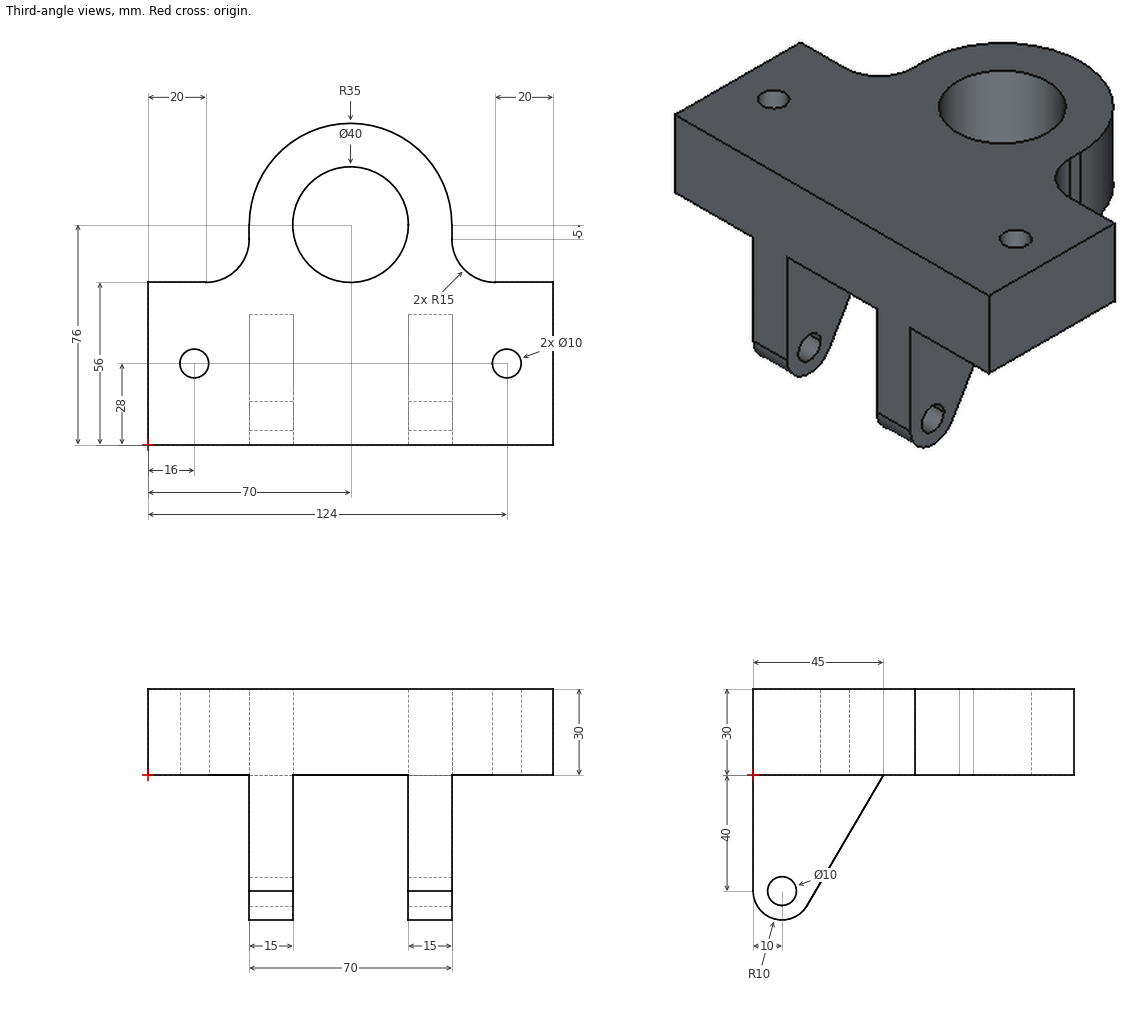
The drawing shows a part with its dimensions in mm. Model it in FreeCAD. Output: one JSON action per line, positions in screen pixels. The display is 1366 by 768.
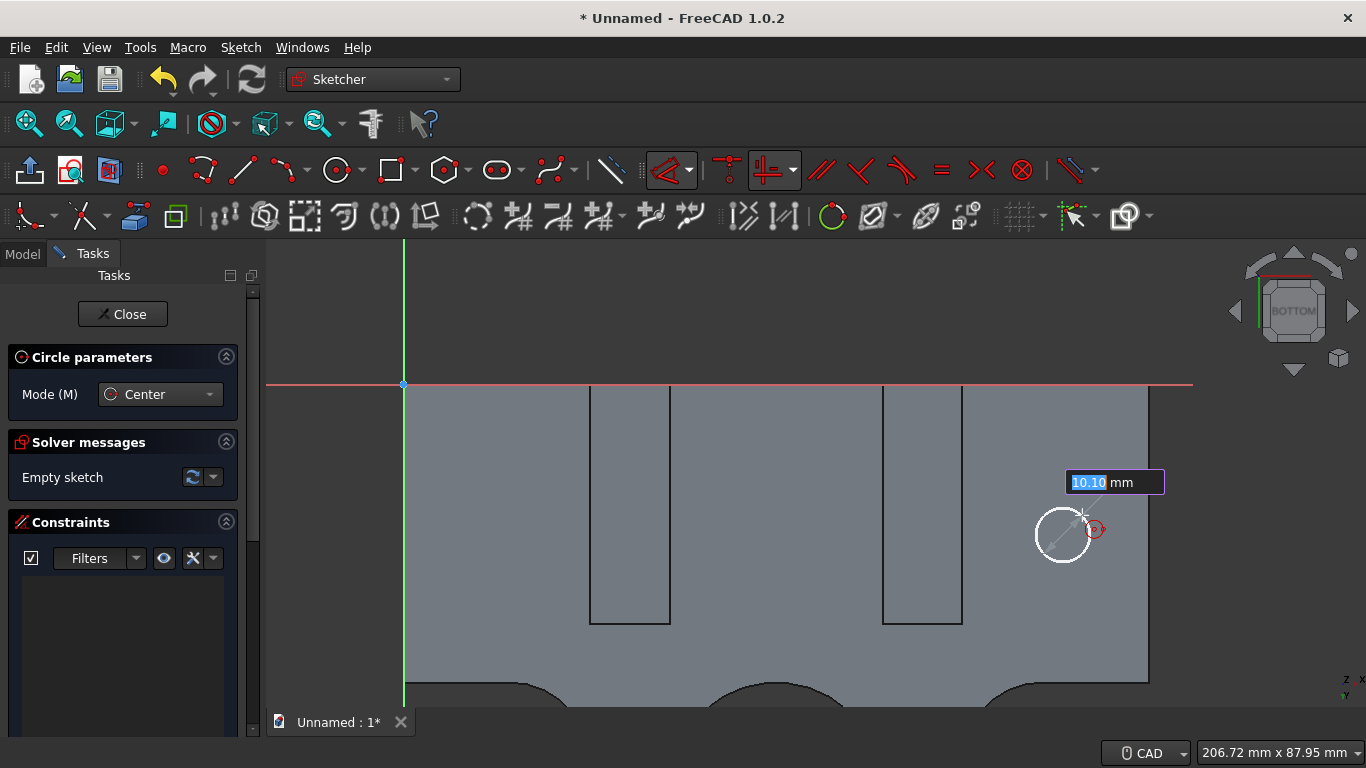
{"action": "type", "text": "10"}
{"action": "key", "text": "Return"}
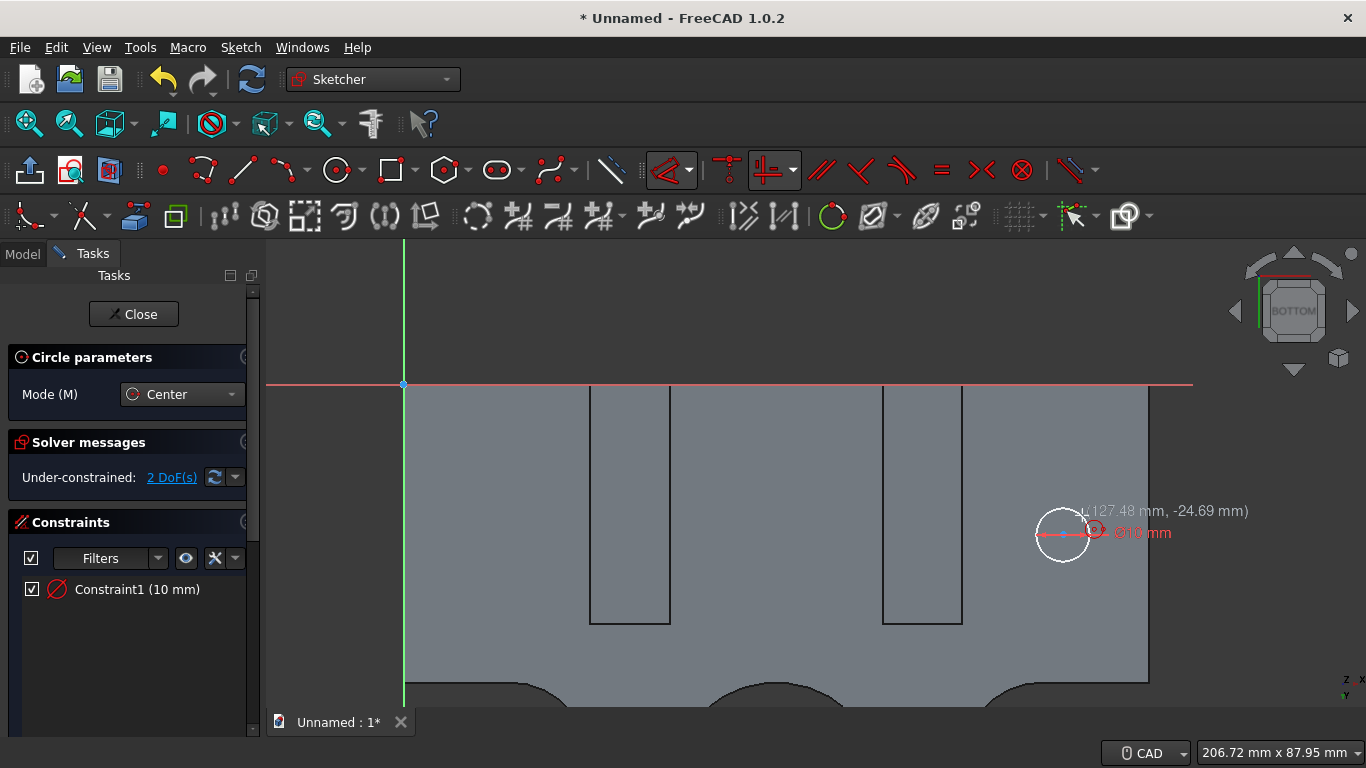
{"action": "left_click", "coordinate": [489, 534]}
{"action": "mouse_move", "coordinate": [508, 515]}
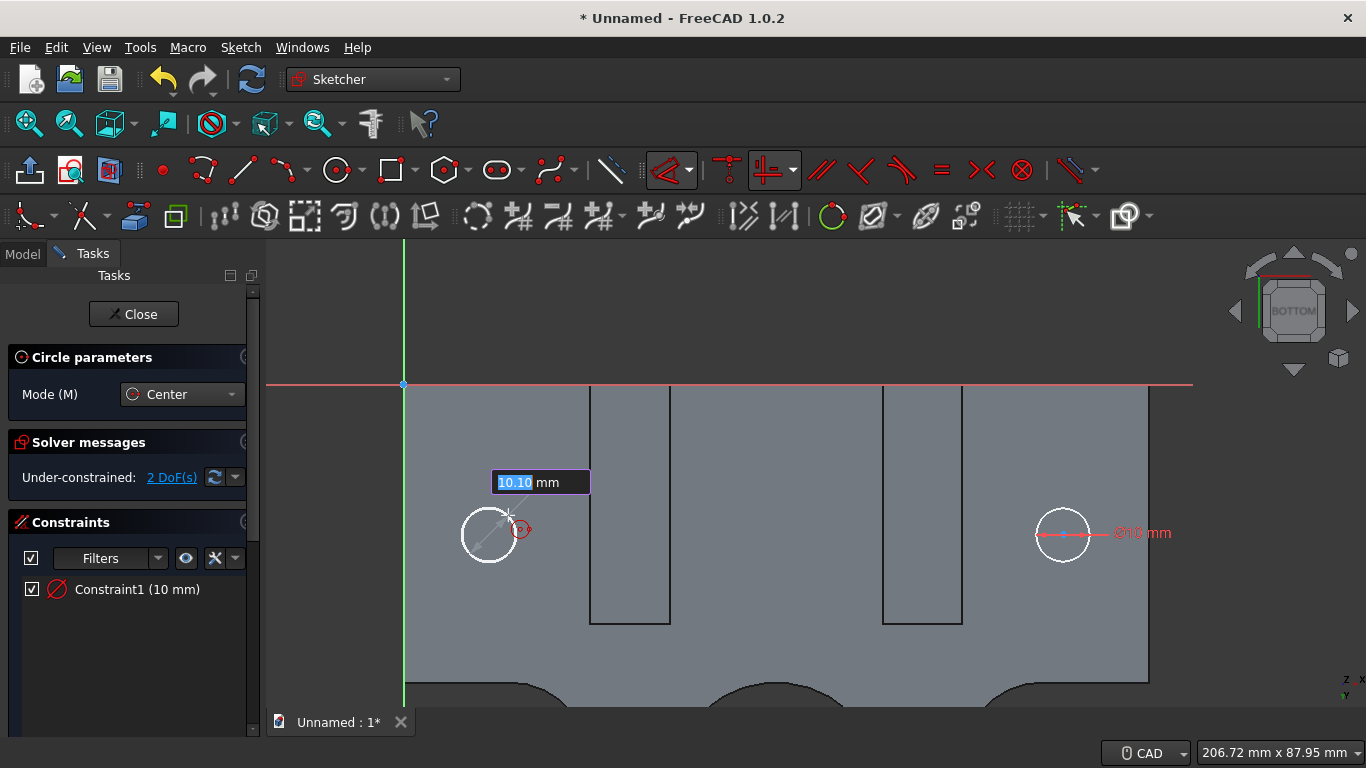
{"action": "type", "text": "10"}
{"action": "key", "text": "Return"}
{"action": "key", "text": "Escape"}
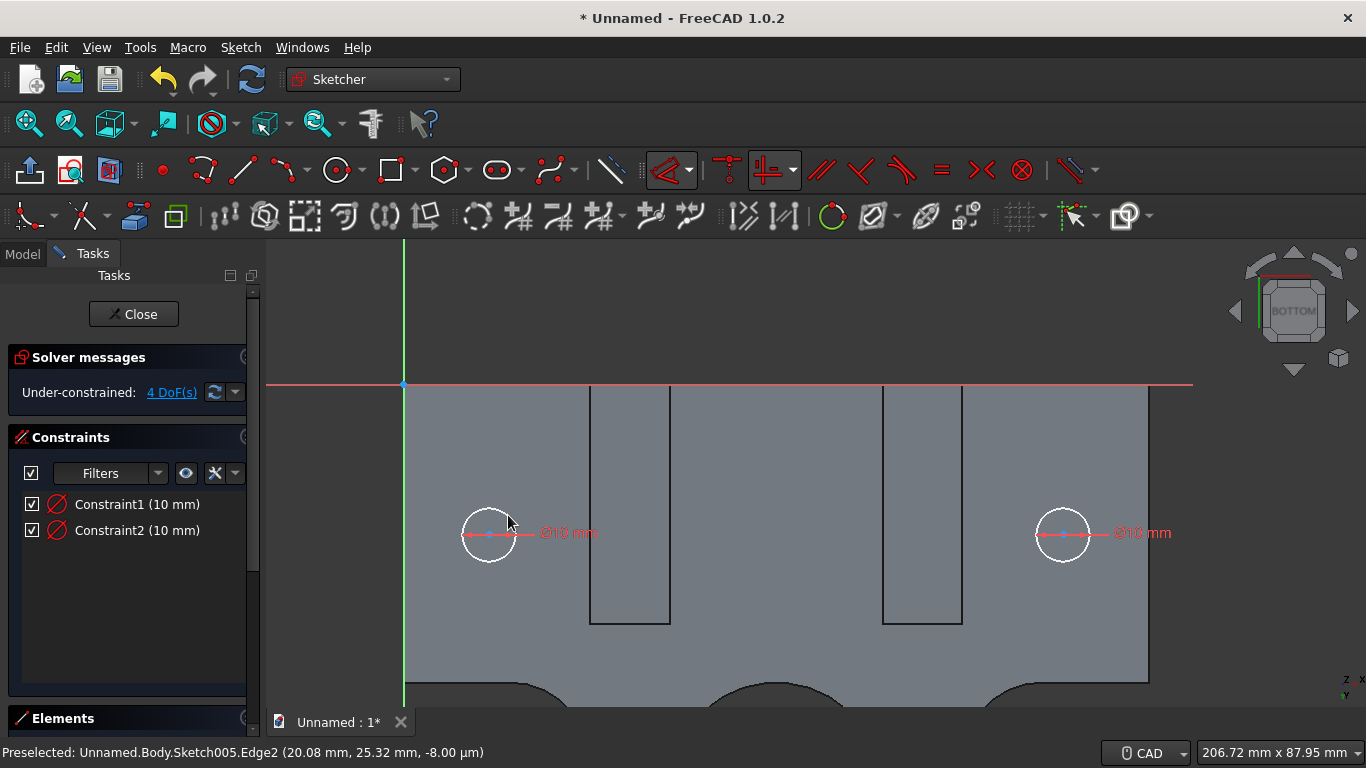
{"action": "left_click", "coordinate": [1063, 535]}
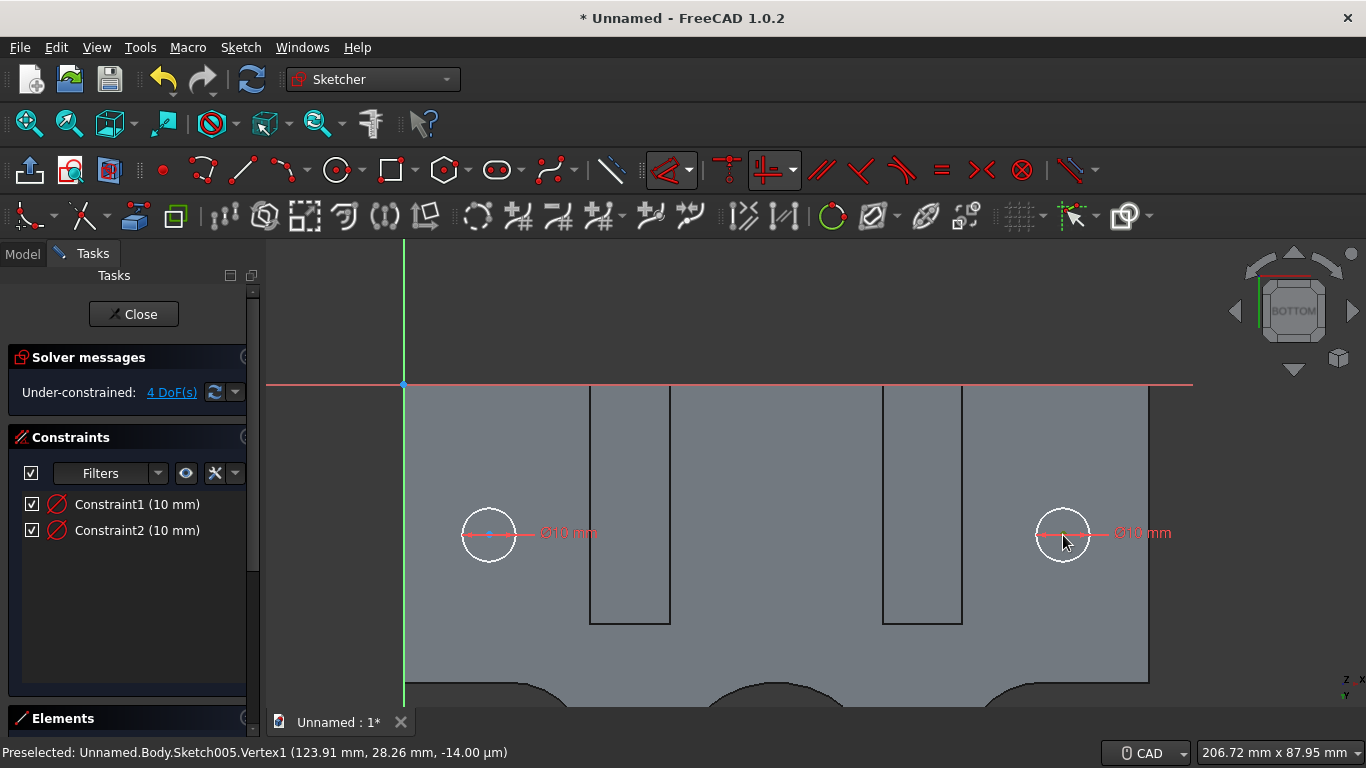
{"action": "left_click", "coordinate": [489, 535]}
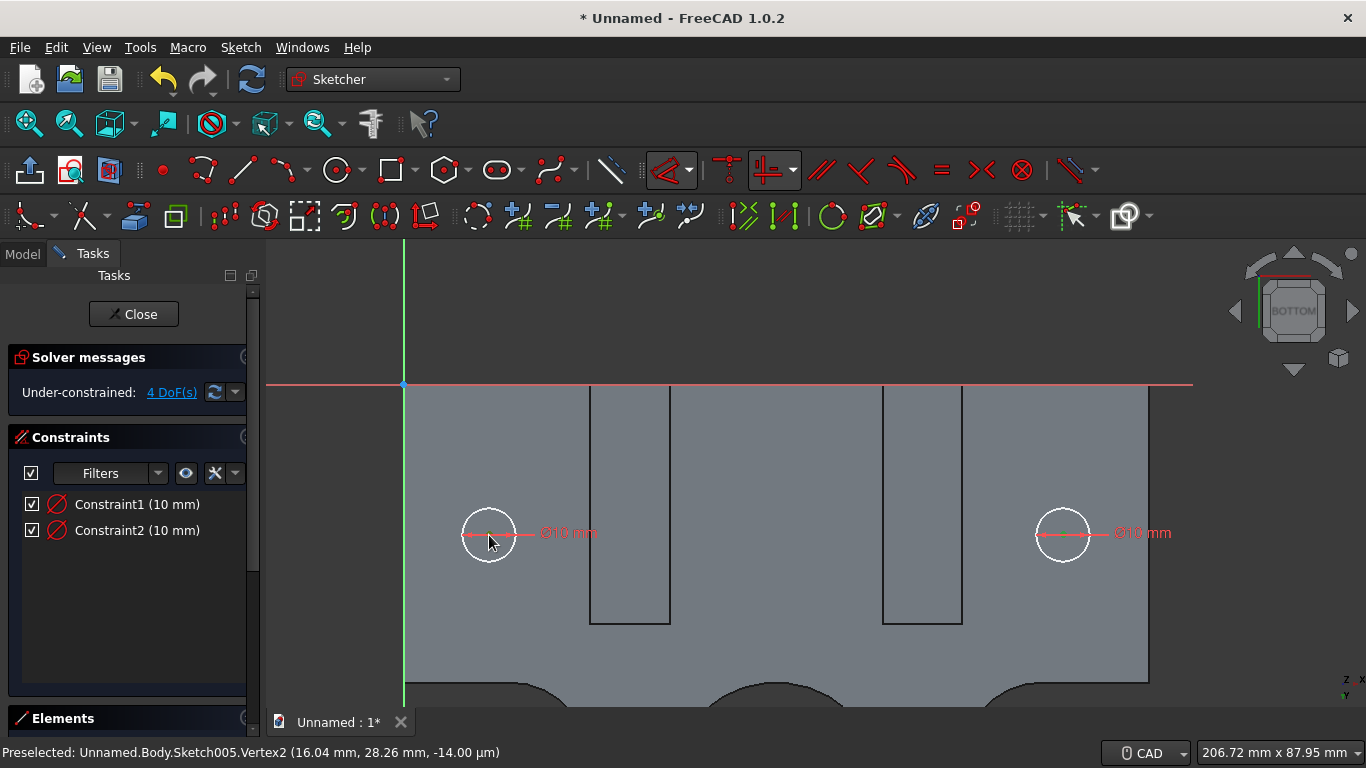
{"action": "key", "text": "h"}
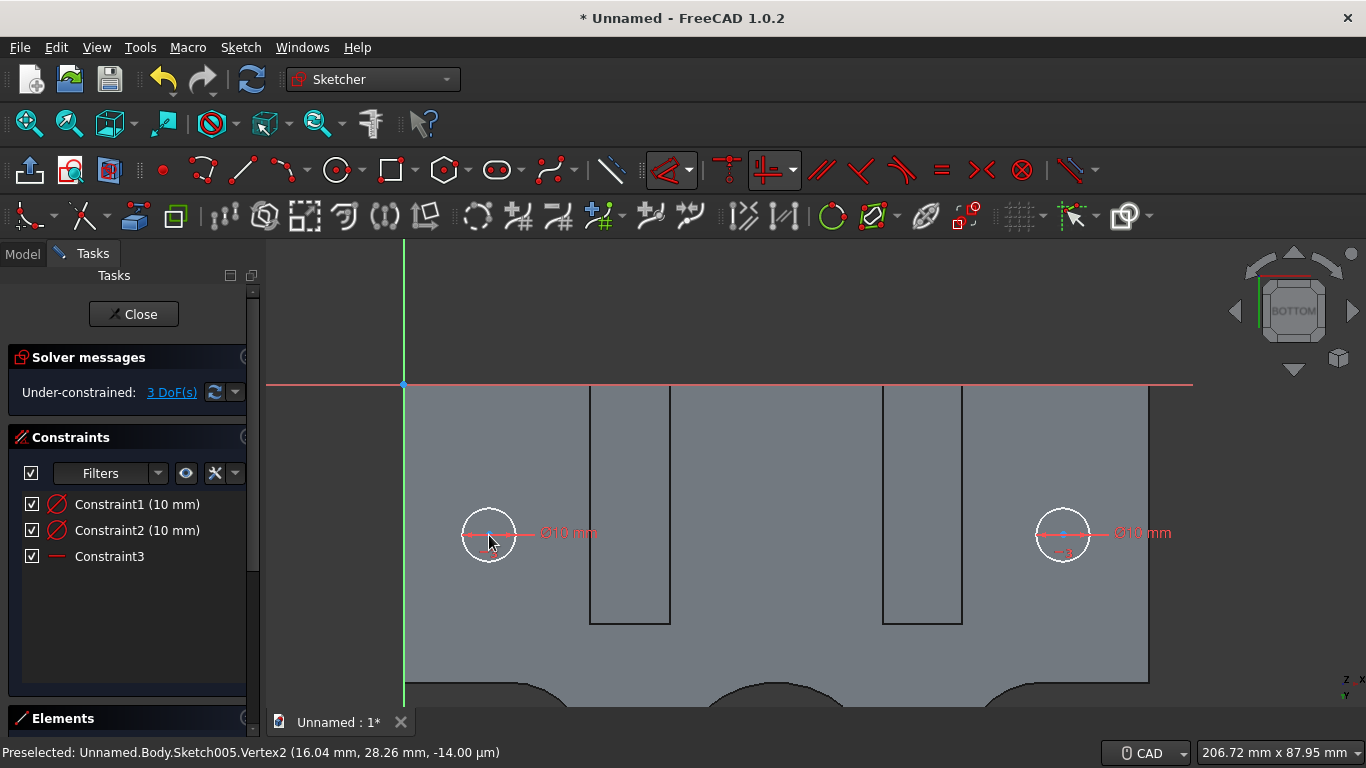
{"action": "left_click", "coordinate": [1063, 535]}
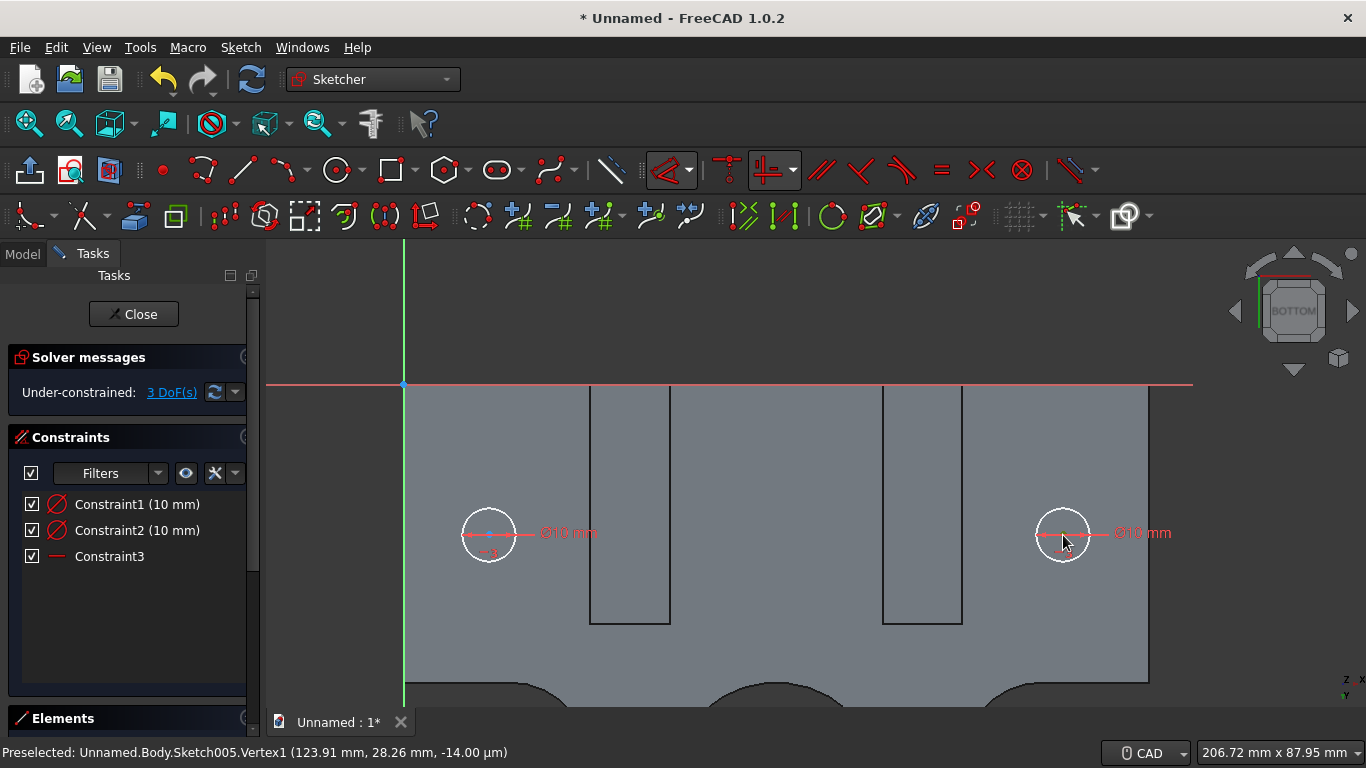
{"action": "left_click", "coordinate": [692, 170]}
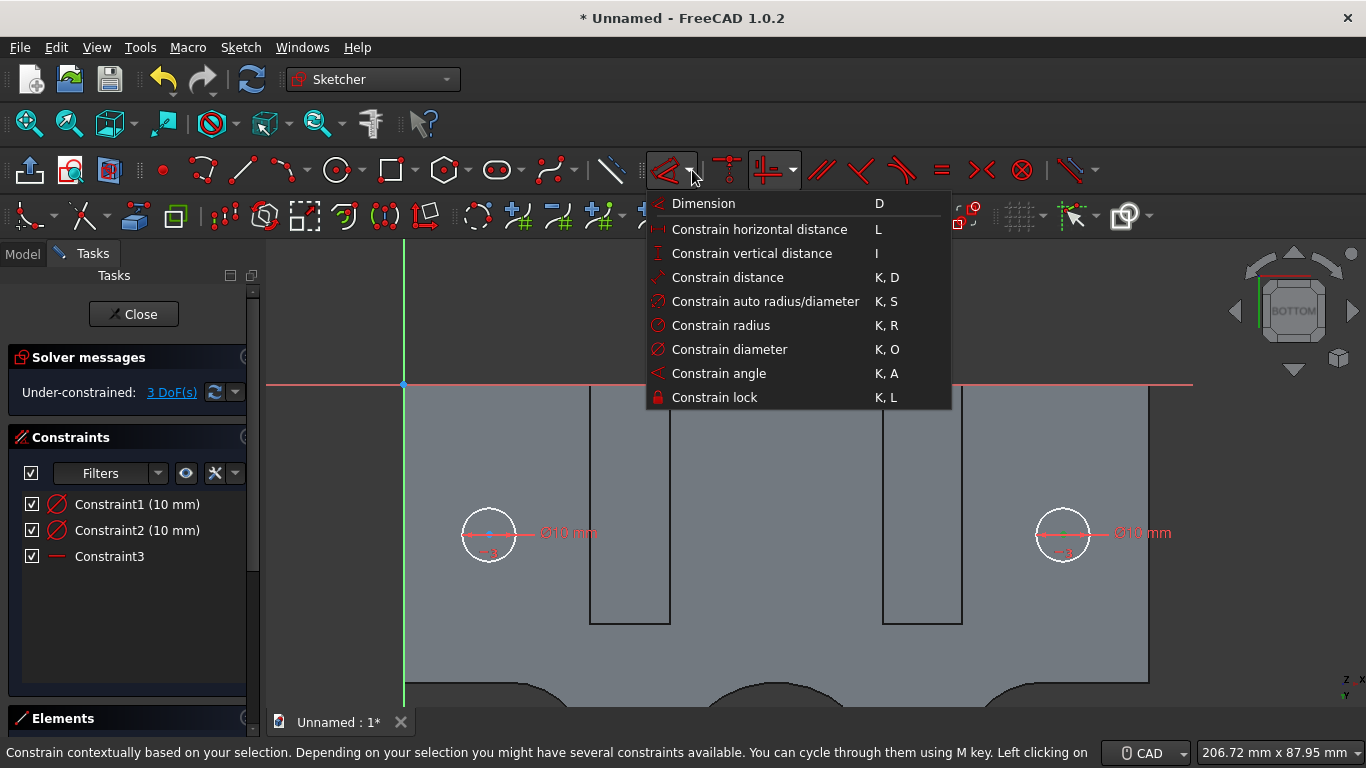
{"action": "left_click", "coordinate": [799, 253]}